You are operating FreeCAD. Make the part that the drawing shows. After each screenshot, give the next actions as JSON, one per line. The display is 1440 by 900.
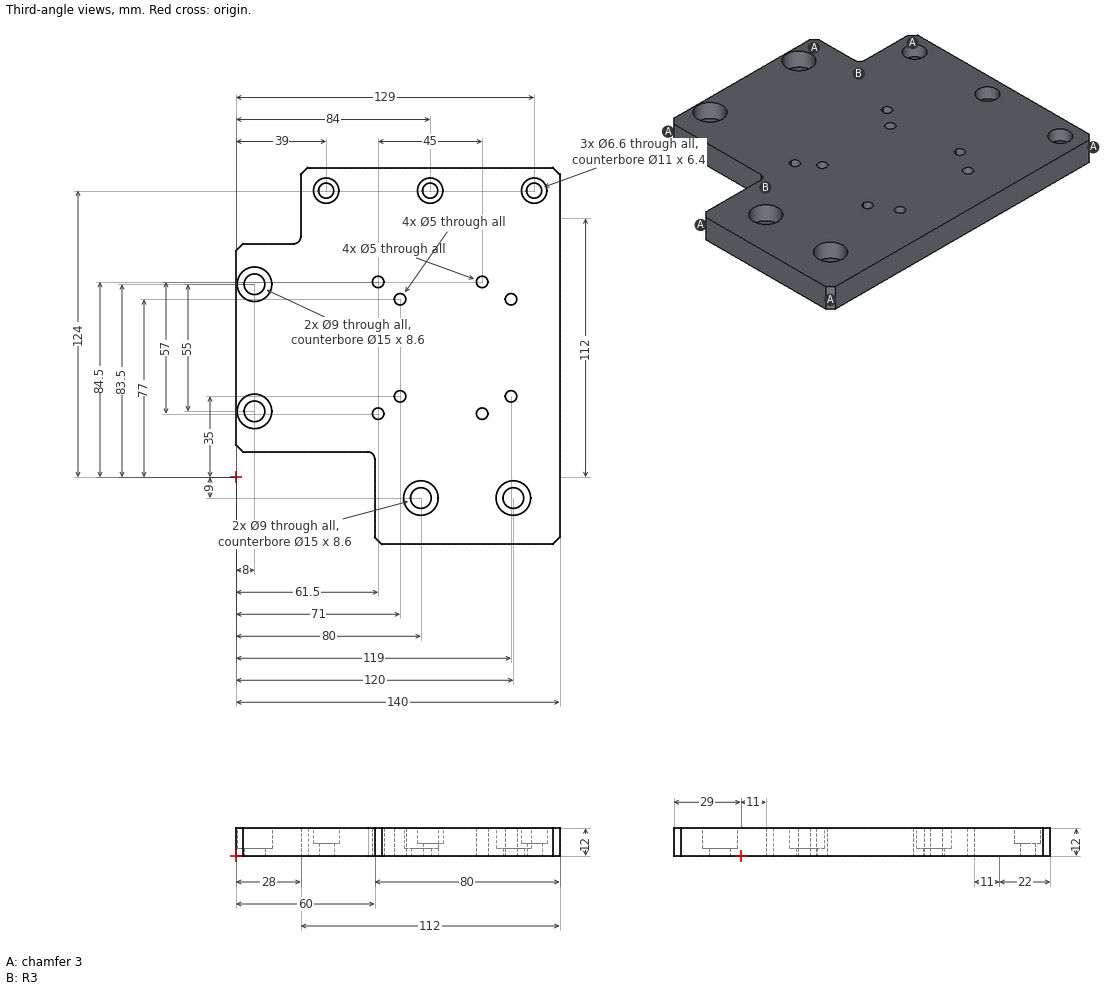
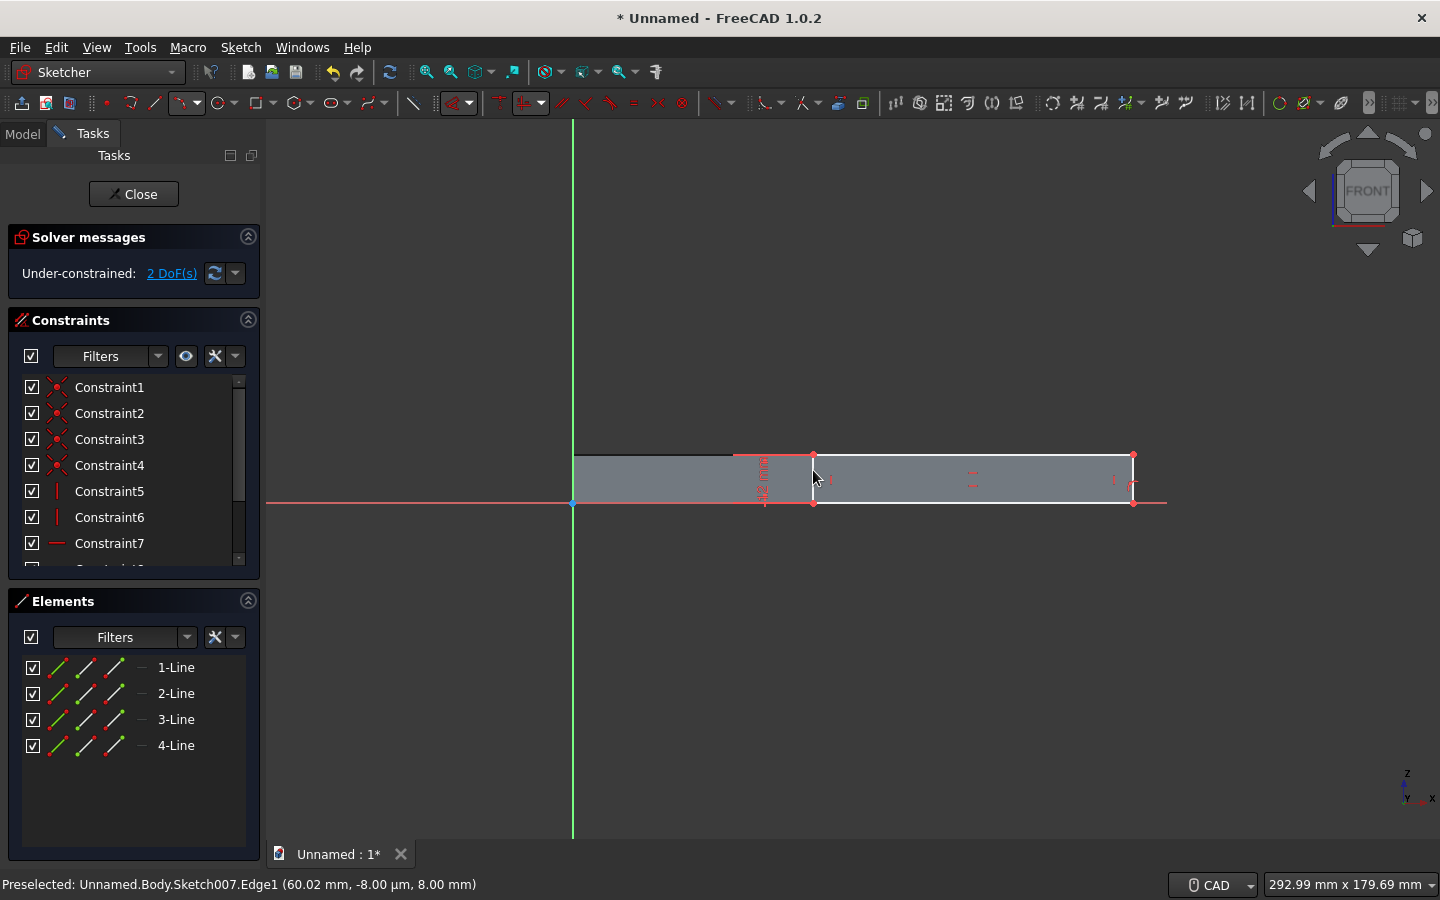
{"action": "left_click", "coordinate": [909, 503]}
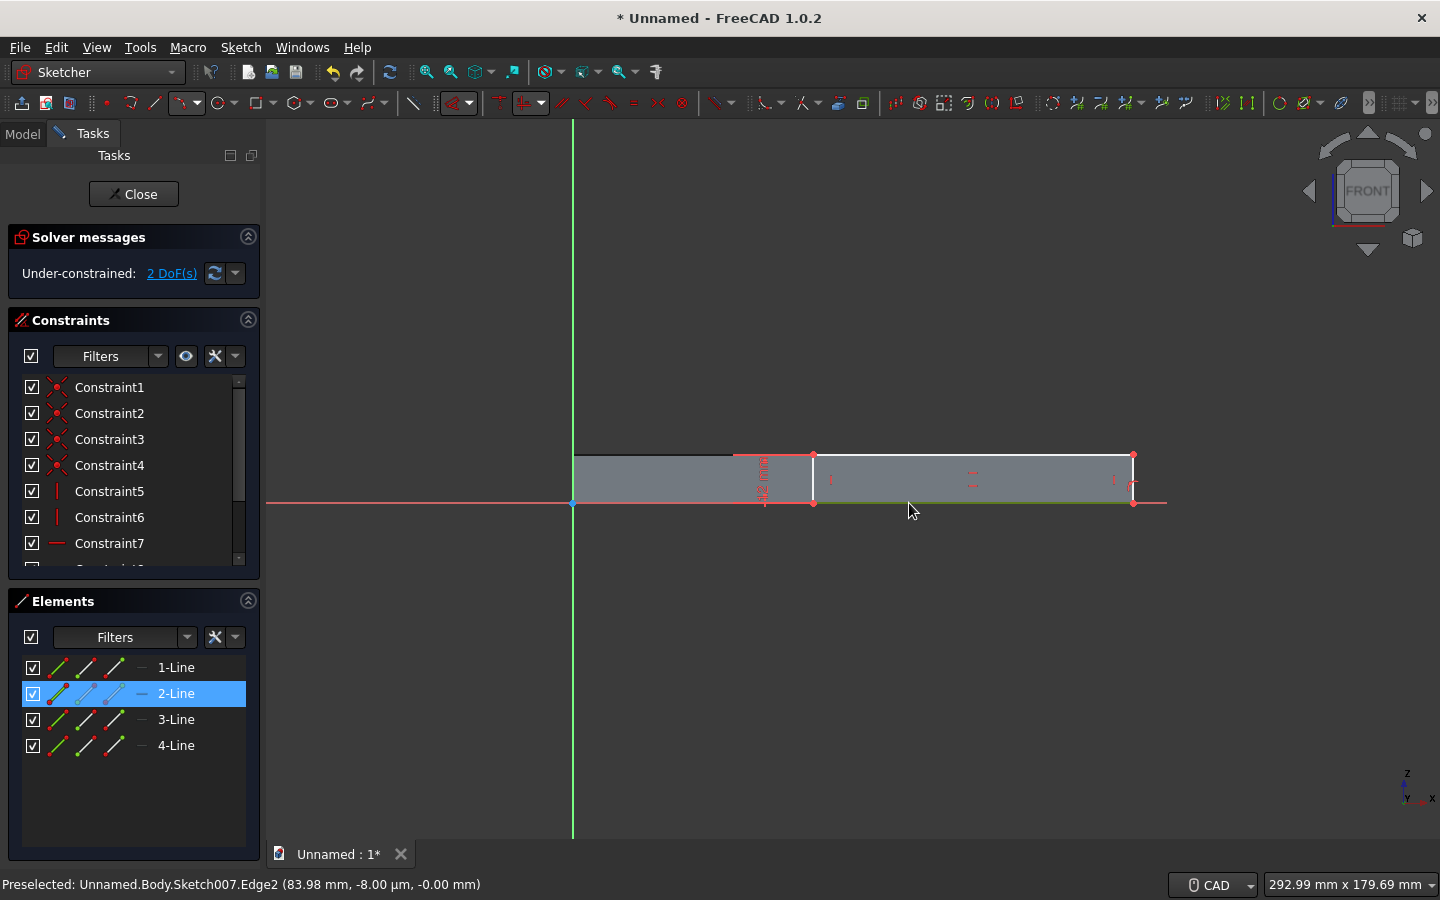
{"action": "key", "text": "l"}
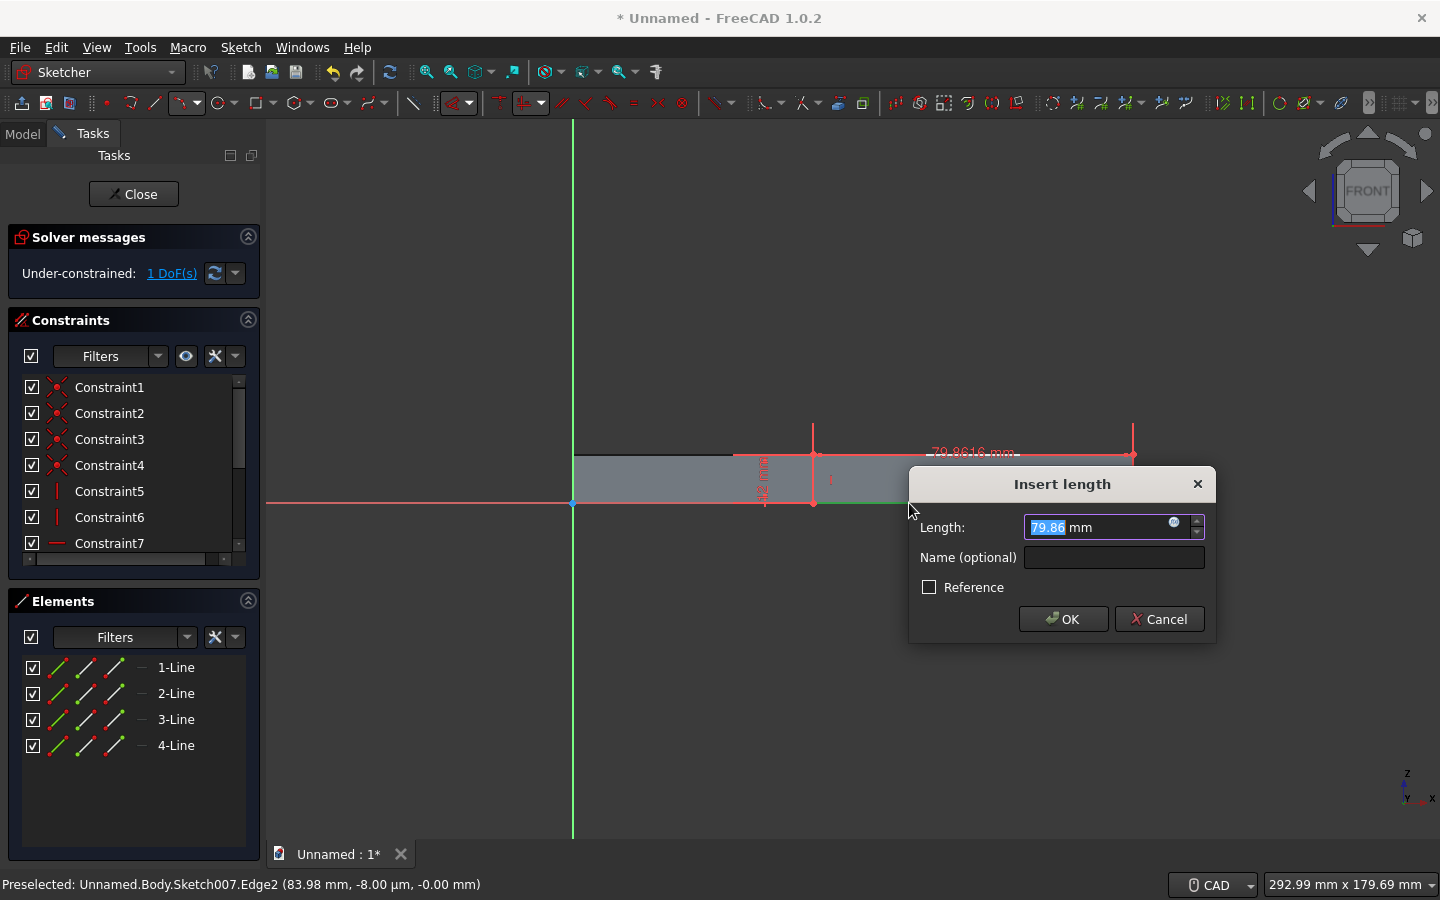
{"action": "type", "text": "80"}
{"action": "key", "text": "Return"}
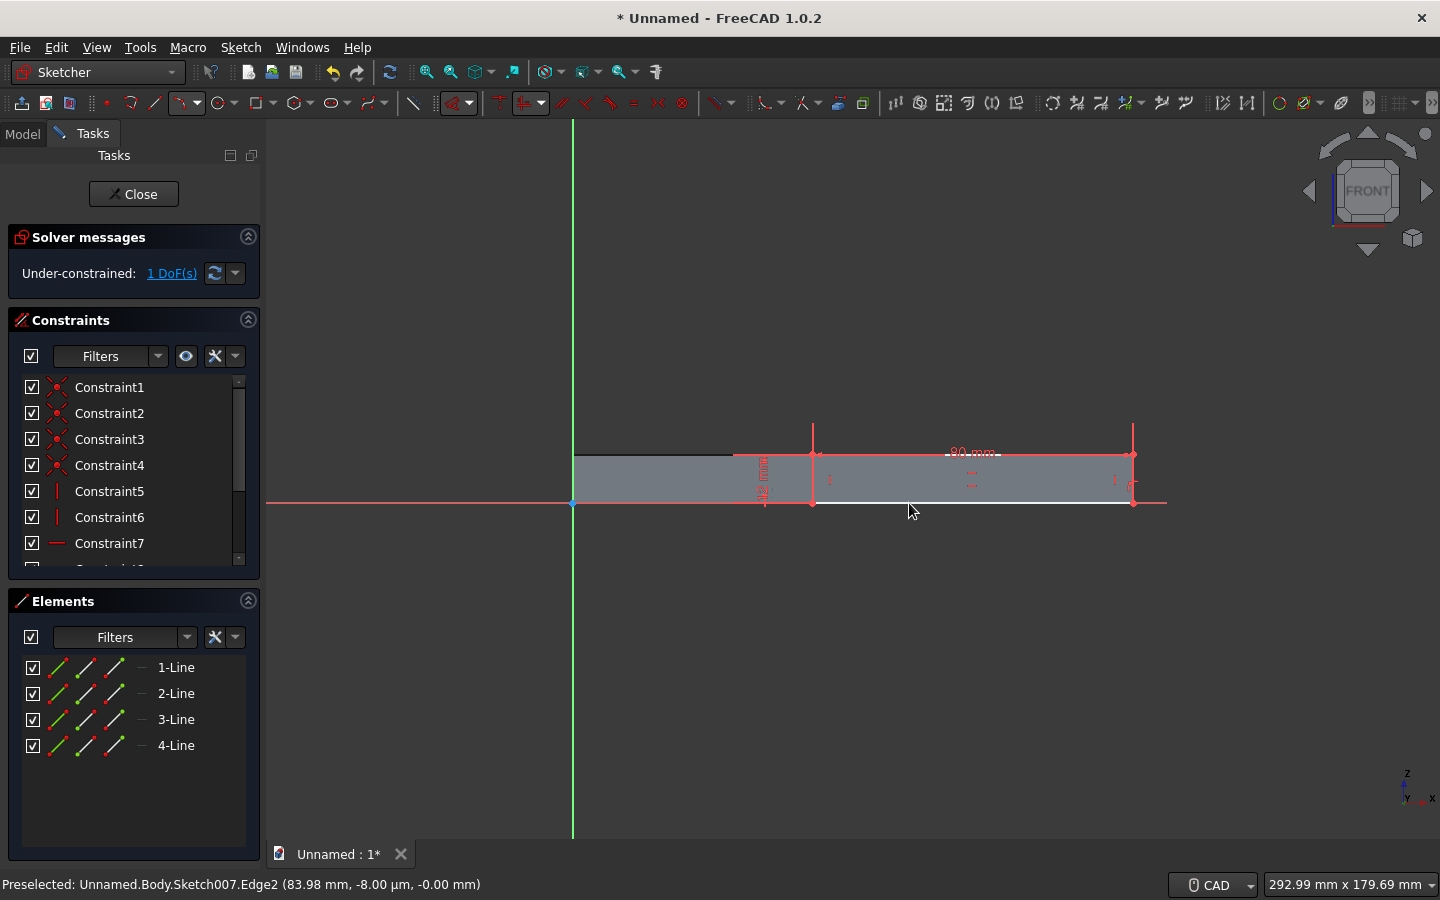
{"action": "left_click", "coordinate": [813, 455]}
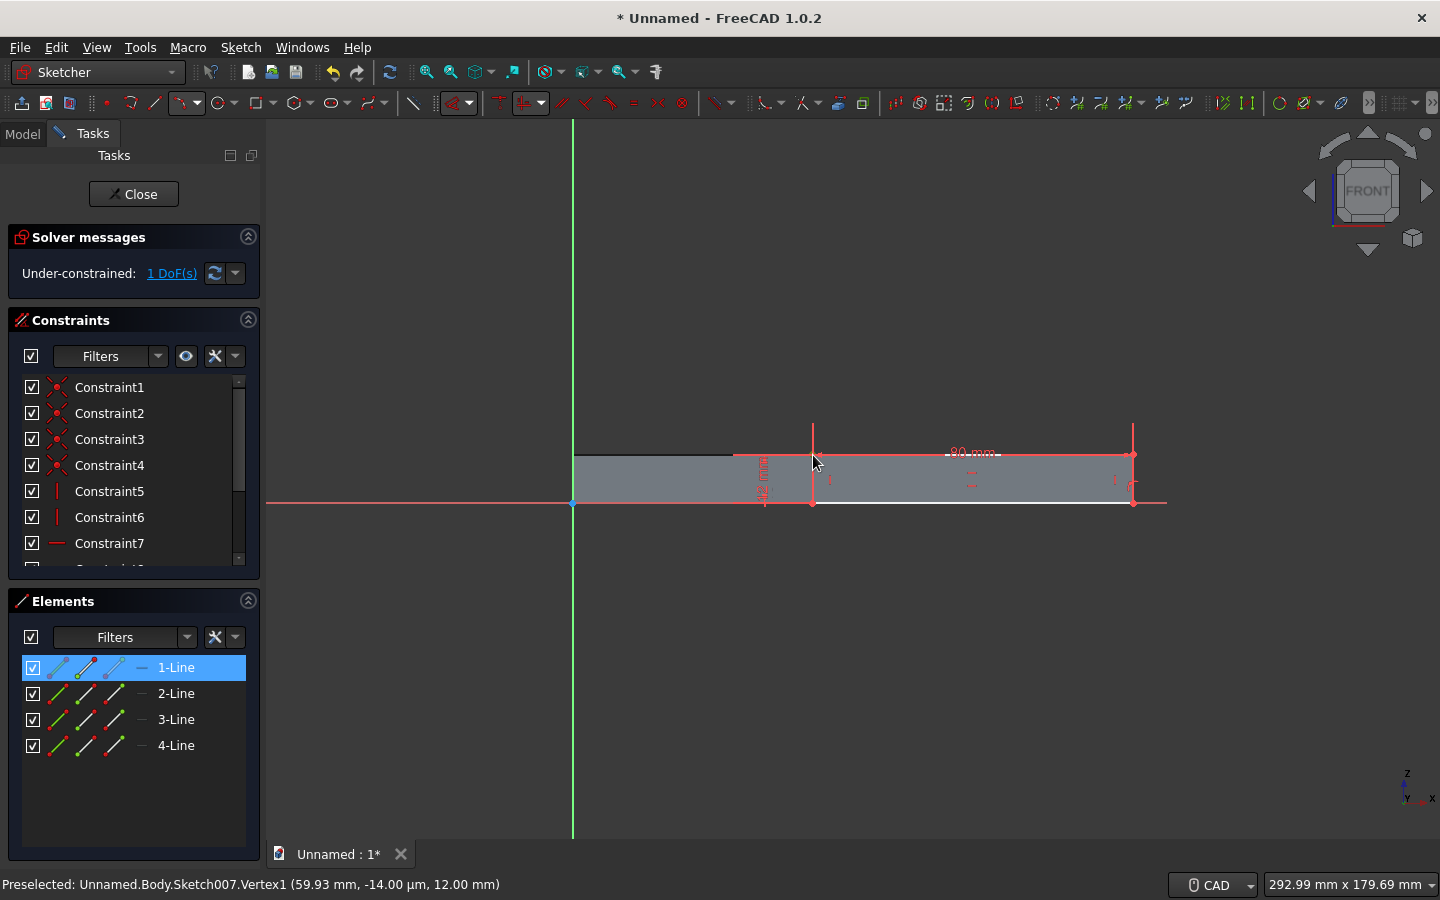
{"action": "key", "text": "l"}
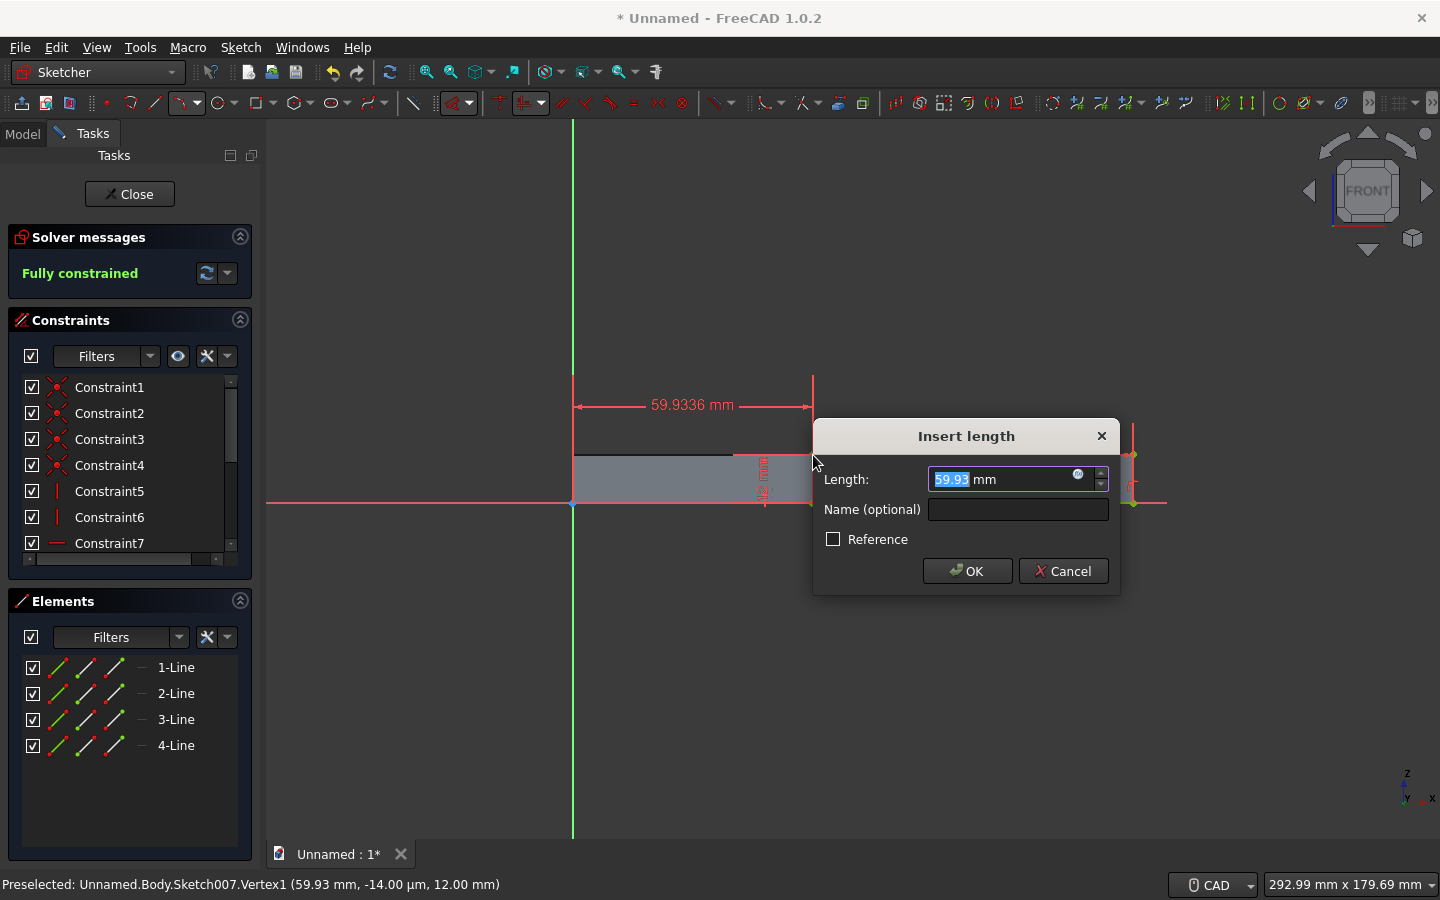
{"action": "type", "text": "60"}
{"action": "key", "text": "Return"}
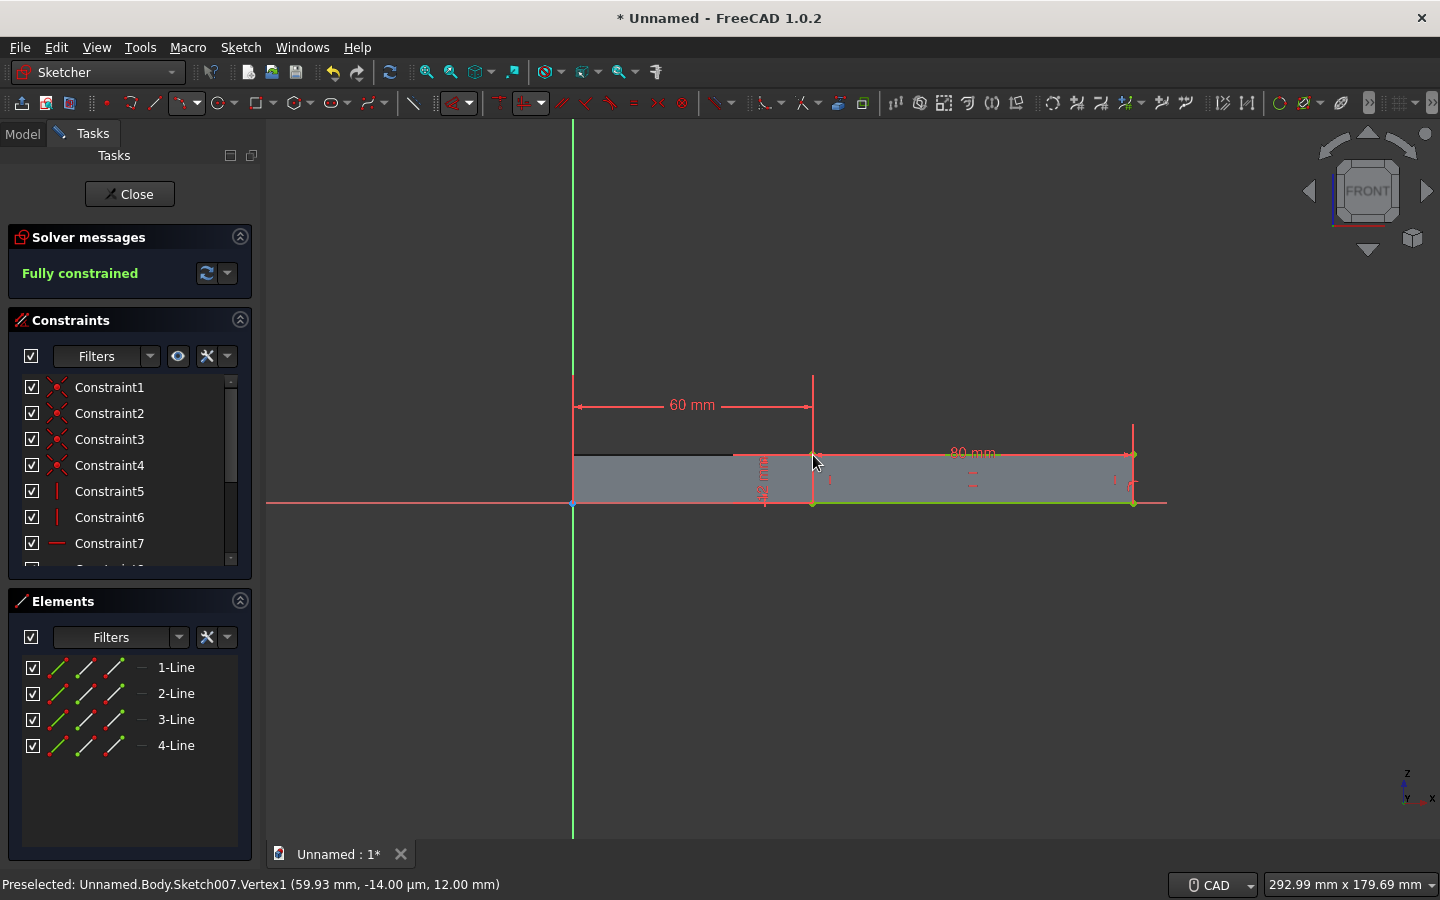
{"action": "left_click", "coordinate": [130, 194]}